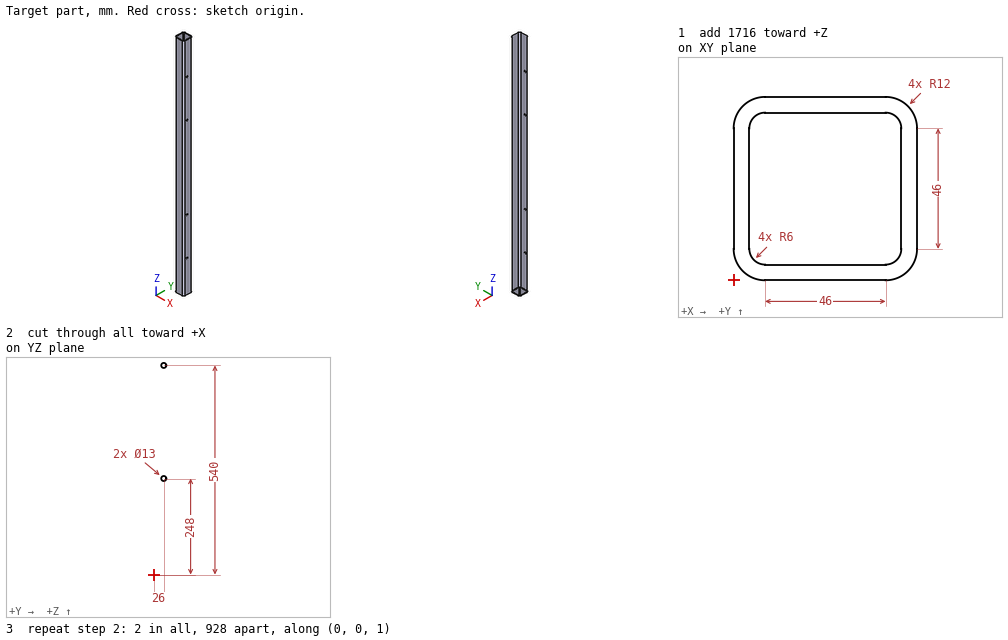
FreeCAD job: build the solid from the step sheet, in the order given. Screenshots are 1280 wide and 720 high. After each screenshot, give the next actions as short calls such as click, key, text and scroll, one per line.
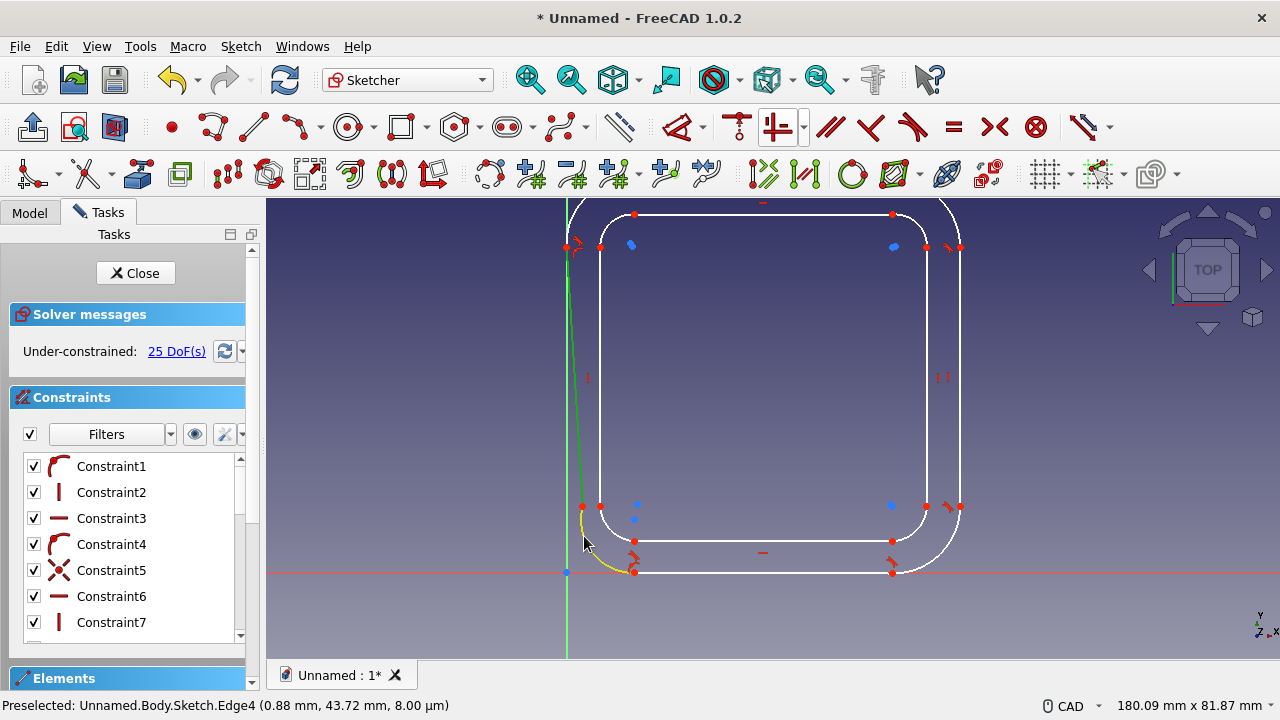
click(583, 535)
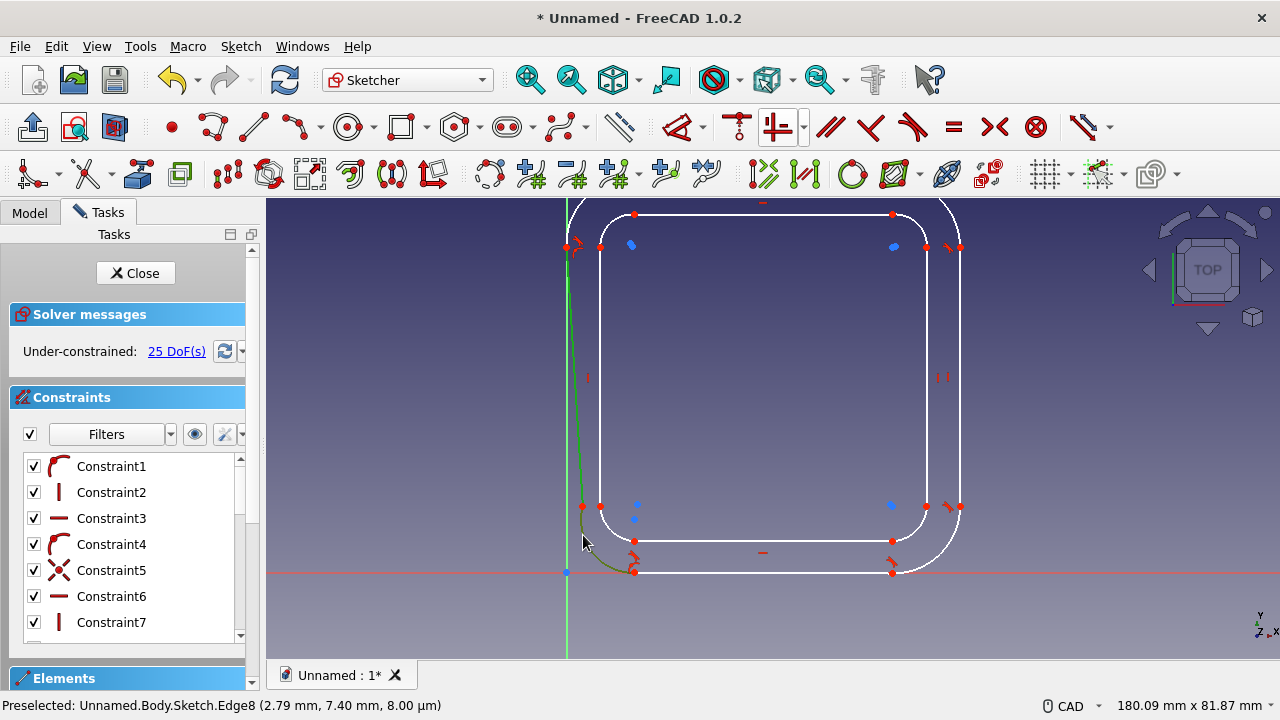
click(913, 128)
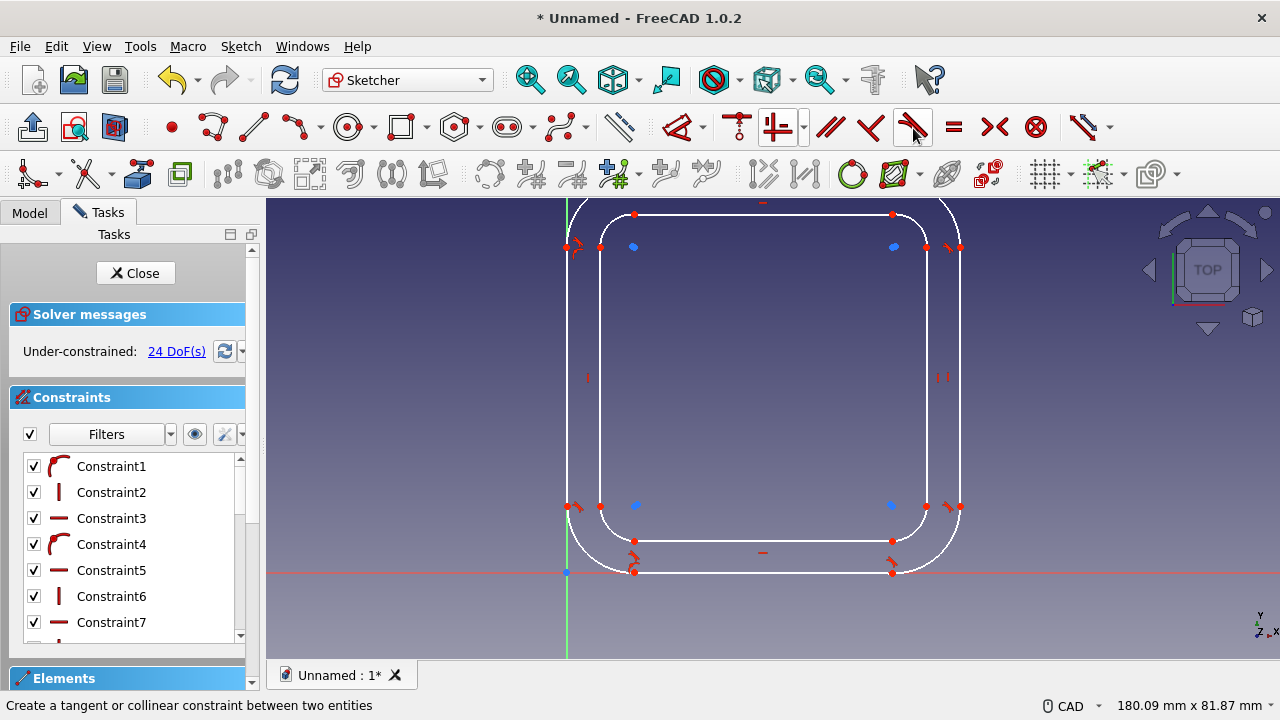
click(815, 541)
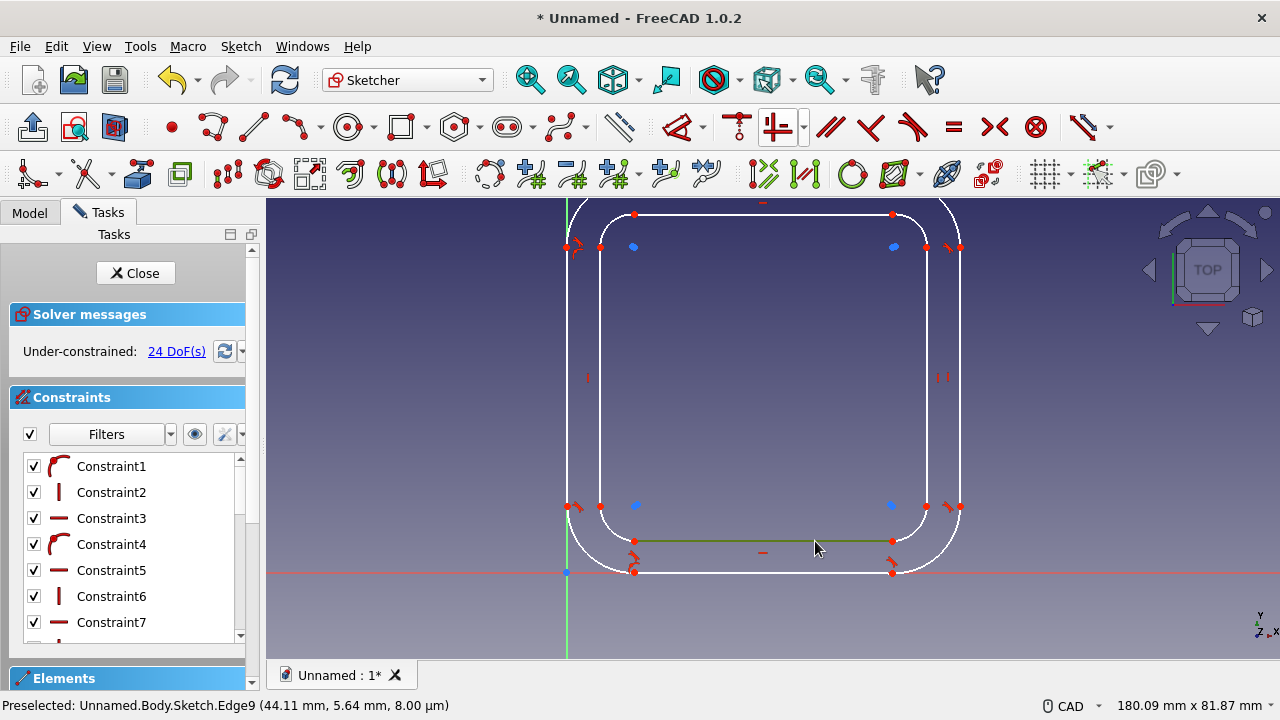
click(605, 522)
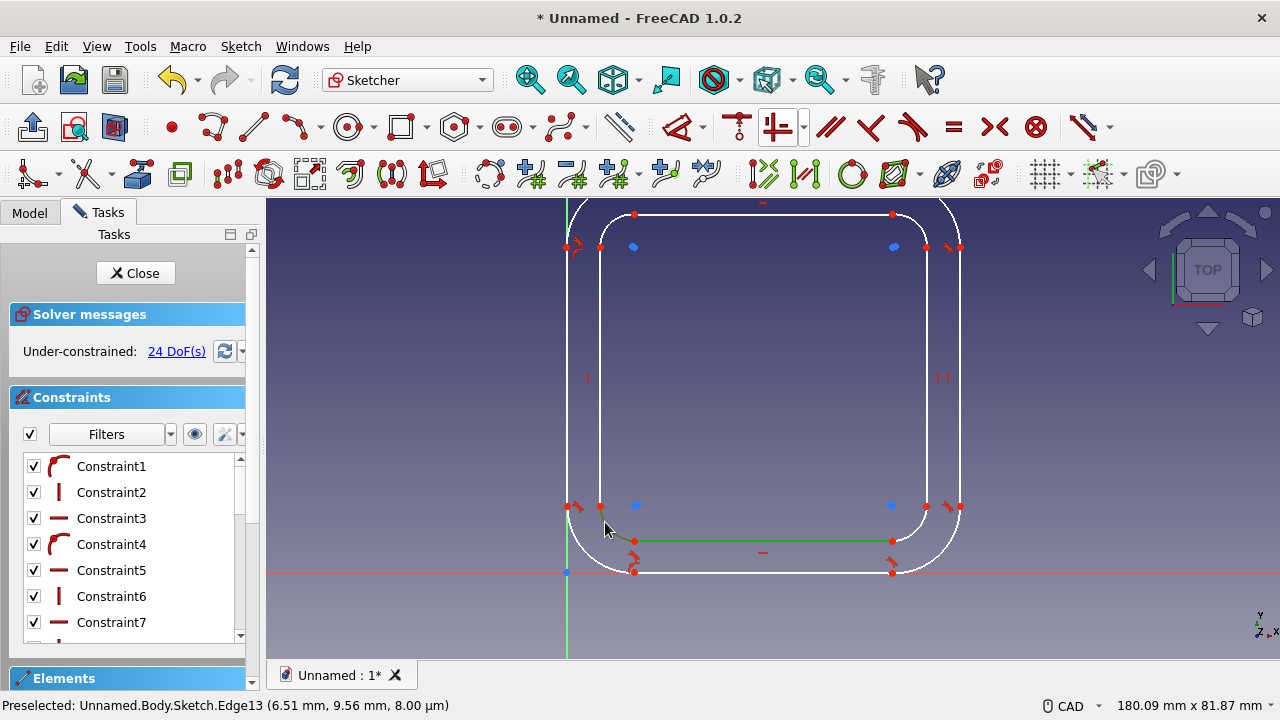
click(913, 128)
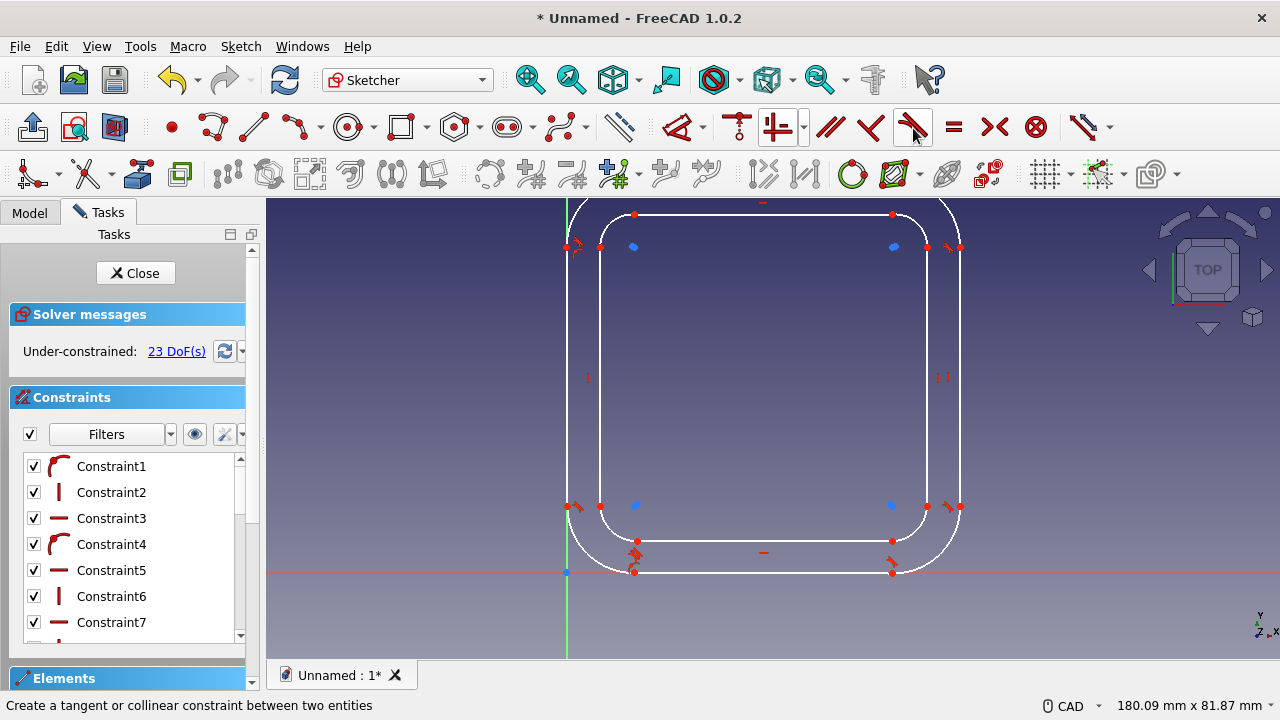
click(816, 541)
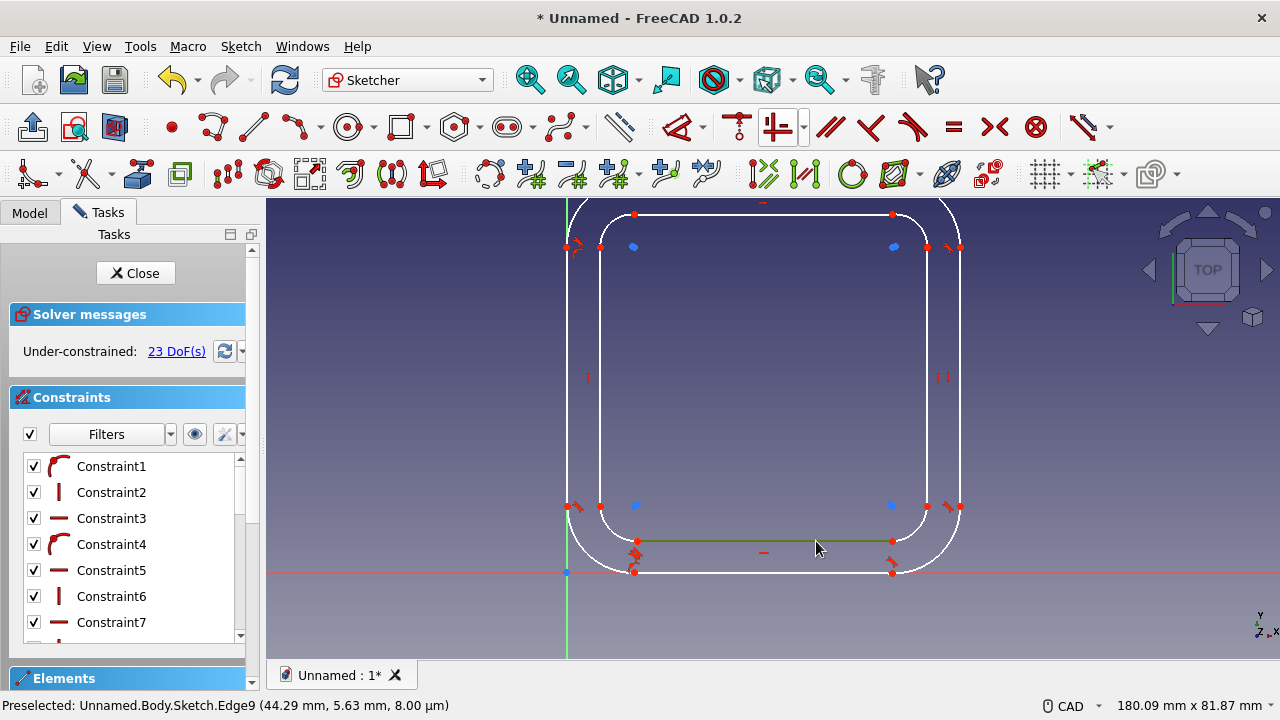
click(908, 537)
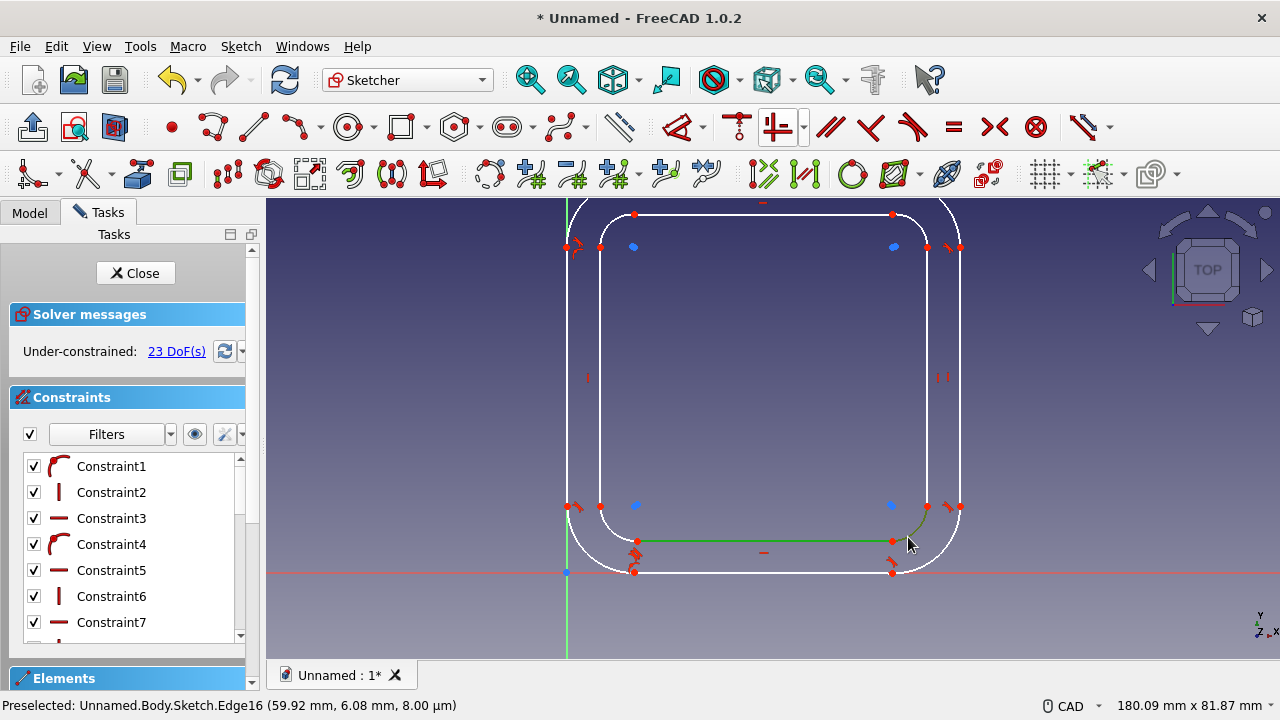
click(913, 128)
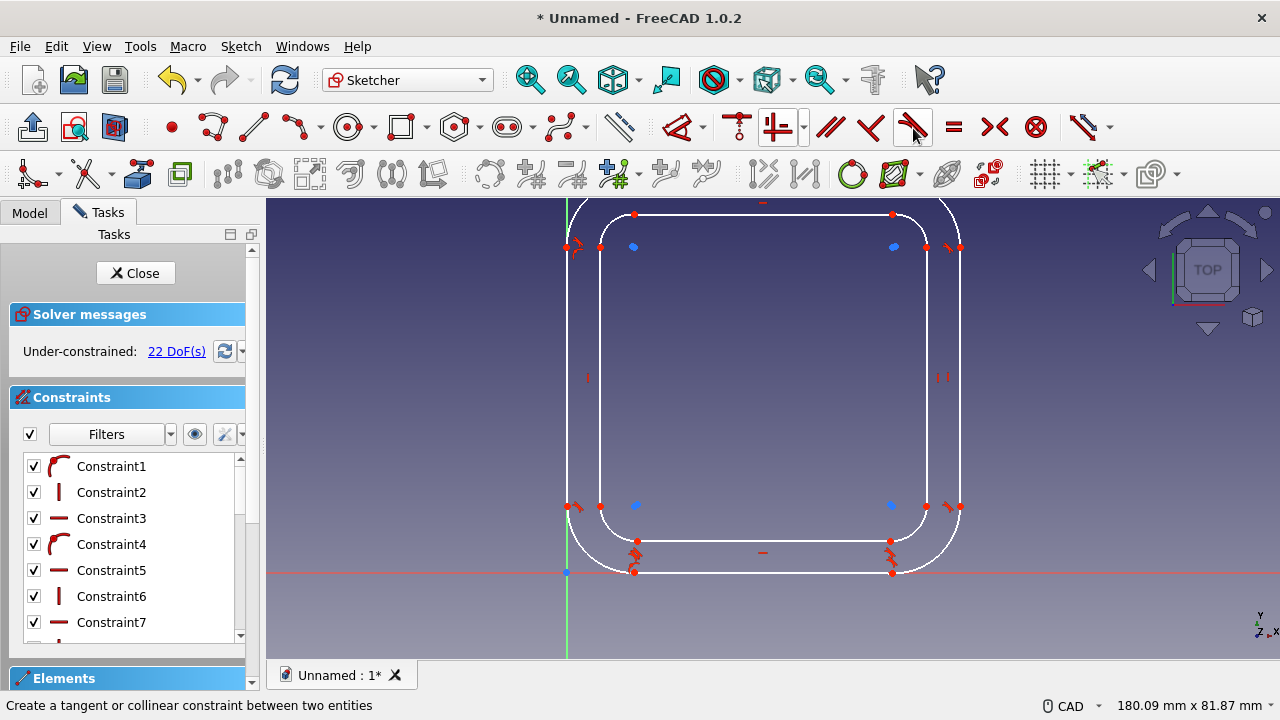
click(600, 429)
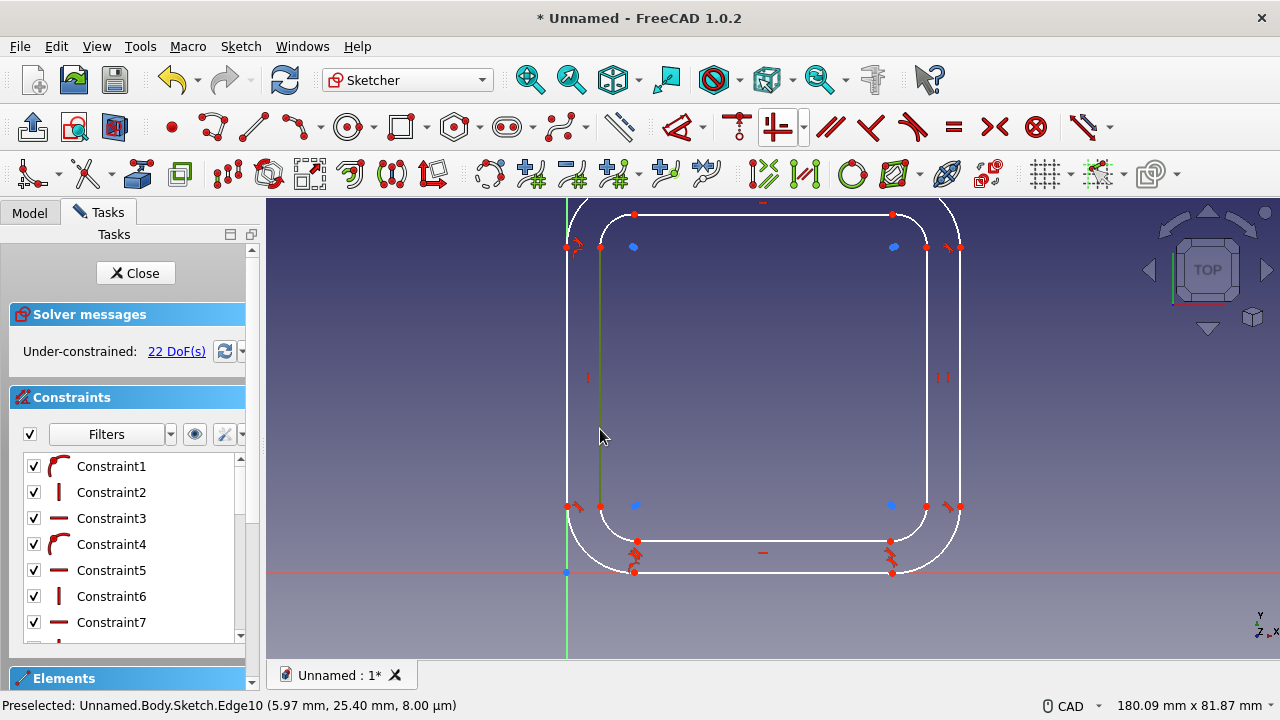
click(605, 523)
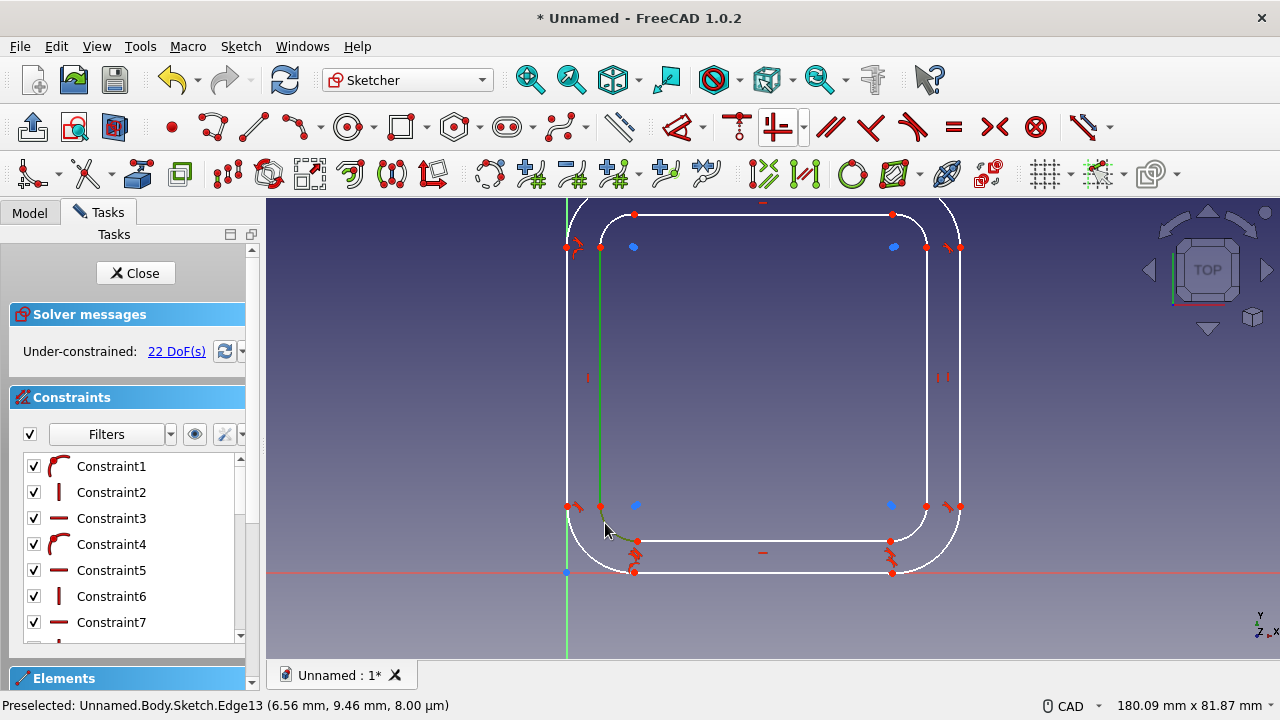
click(913, 128)